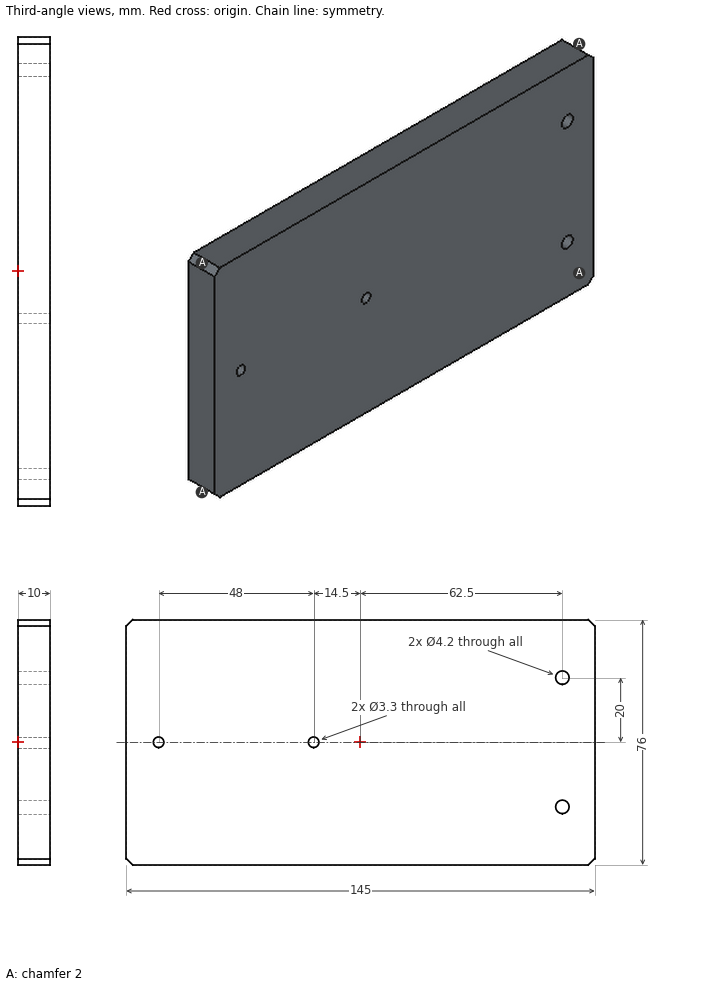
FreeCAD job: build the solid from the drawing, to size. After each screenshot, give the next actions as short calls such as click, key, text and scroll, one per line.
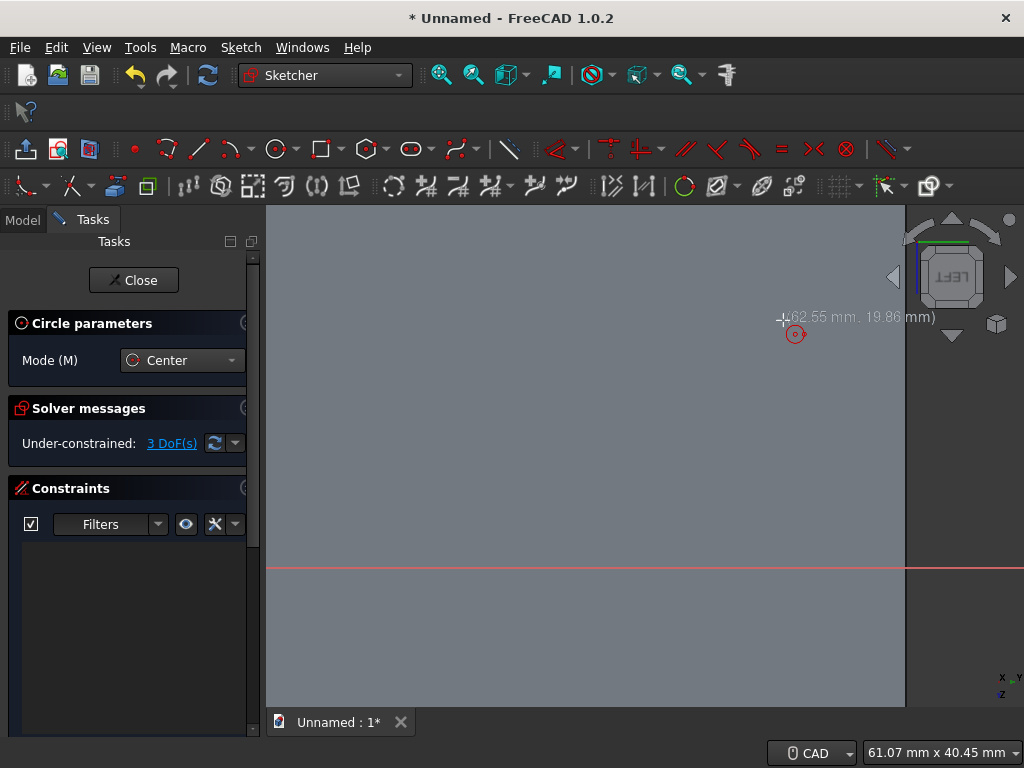
click(782, 320)
click(800, 301)
key(Escape)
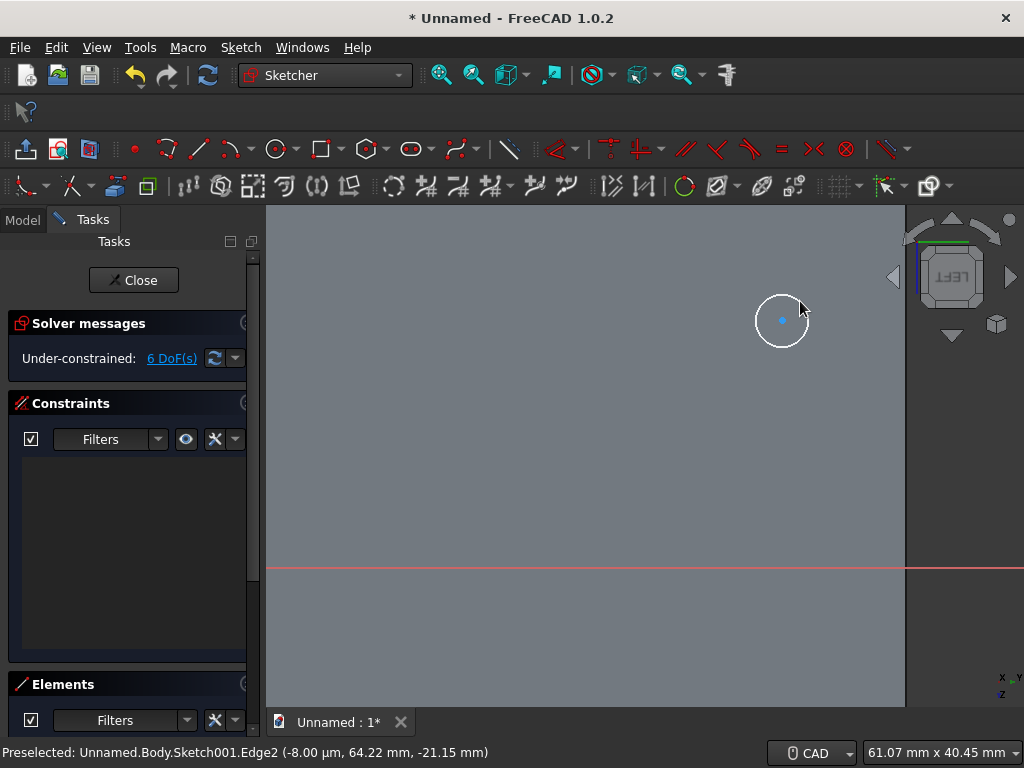
scroll(783, 320, down, 3)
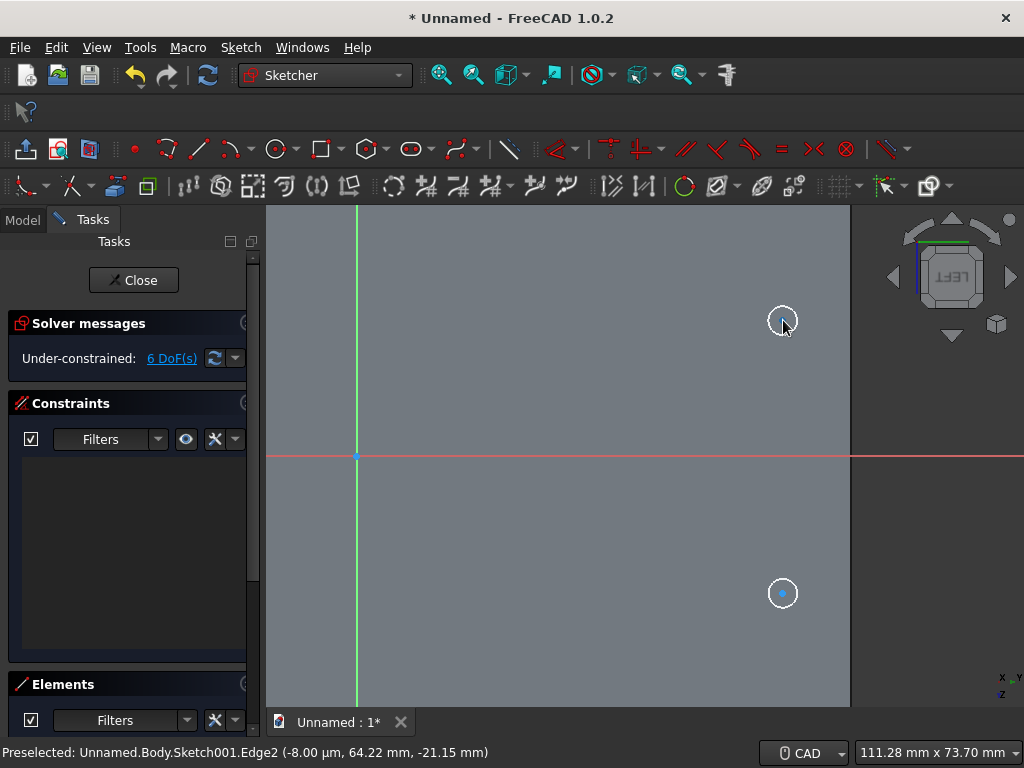
click(793, 583)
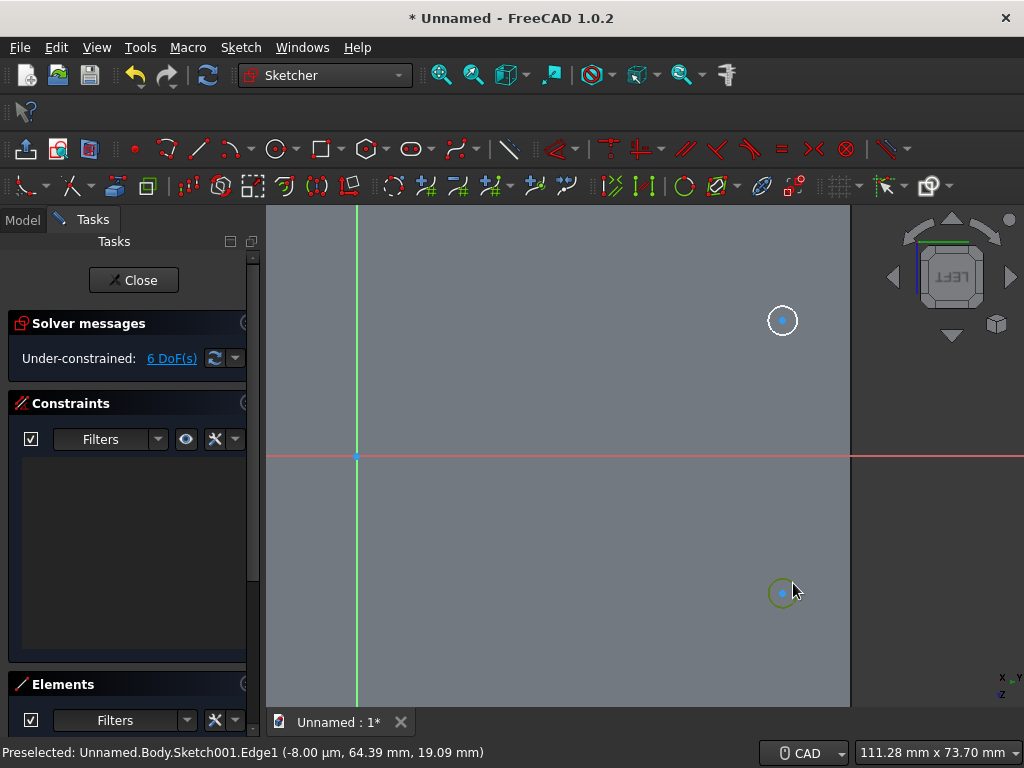
click(793, 310)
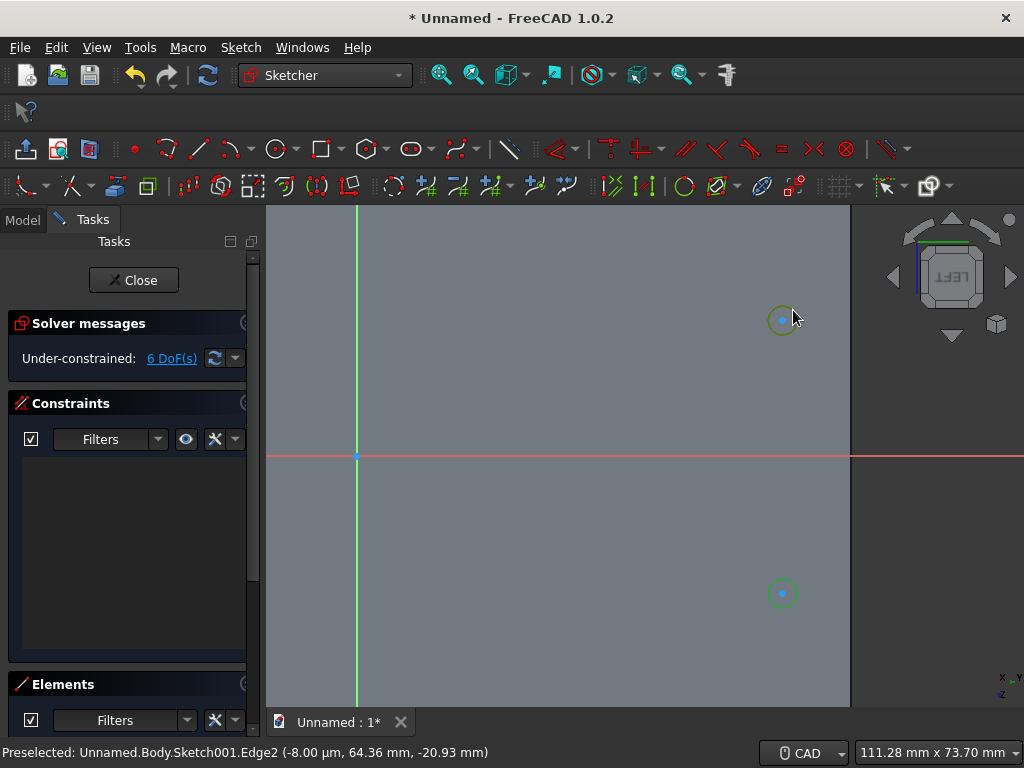
key(e)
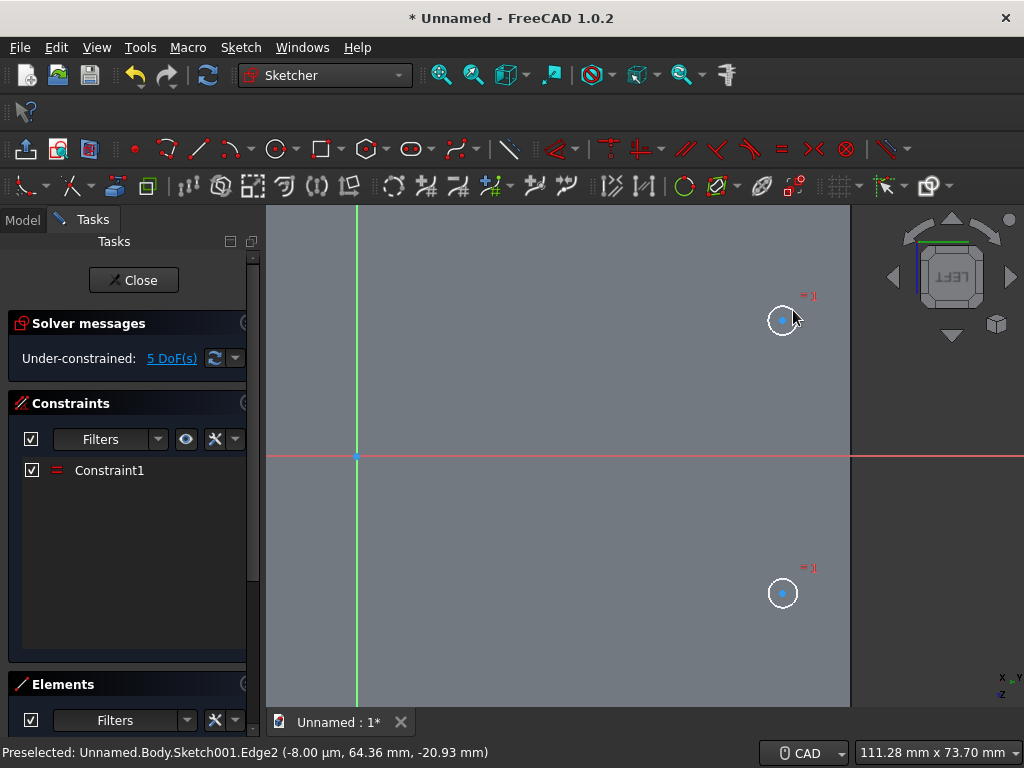
click(783, 593)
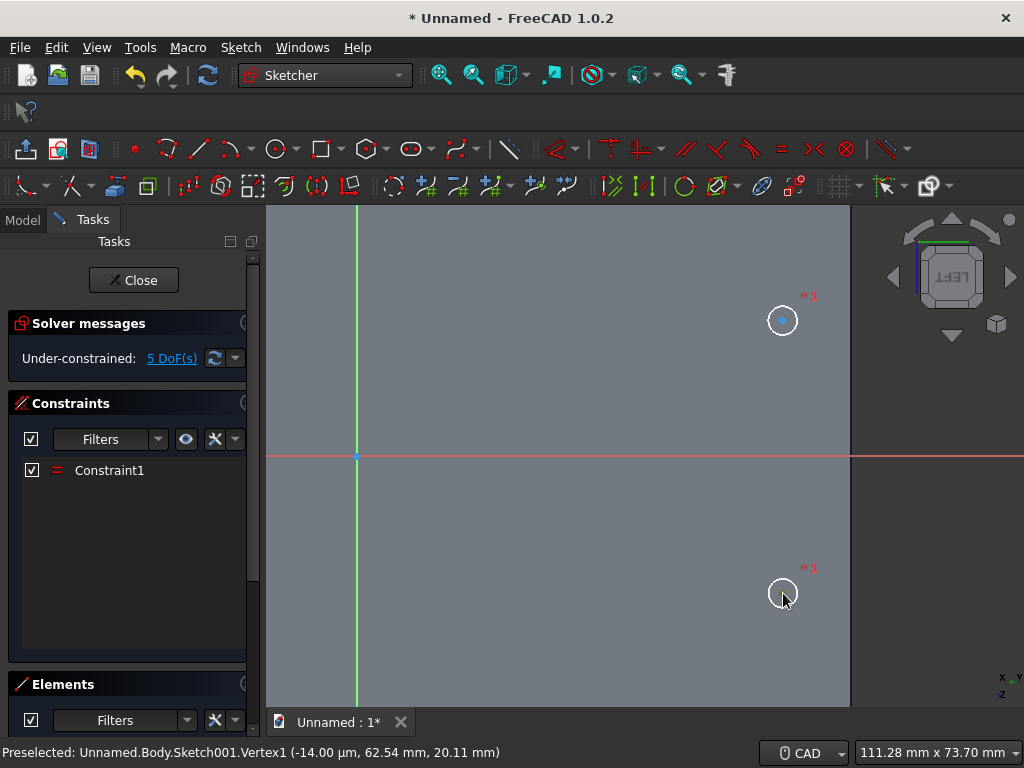
click(783, 321)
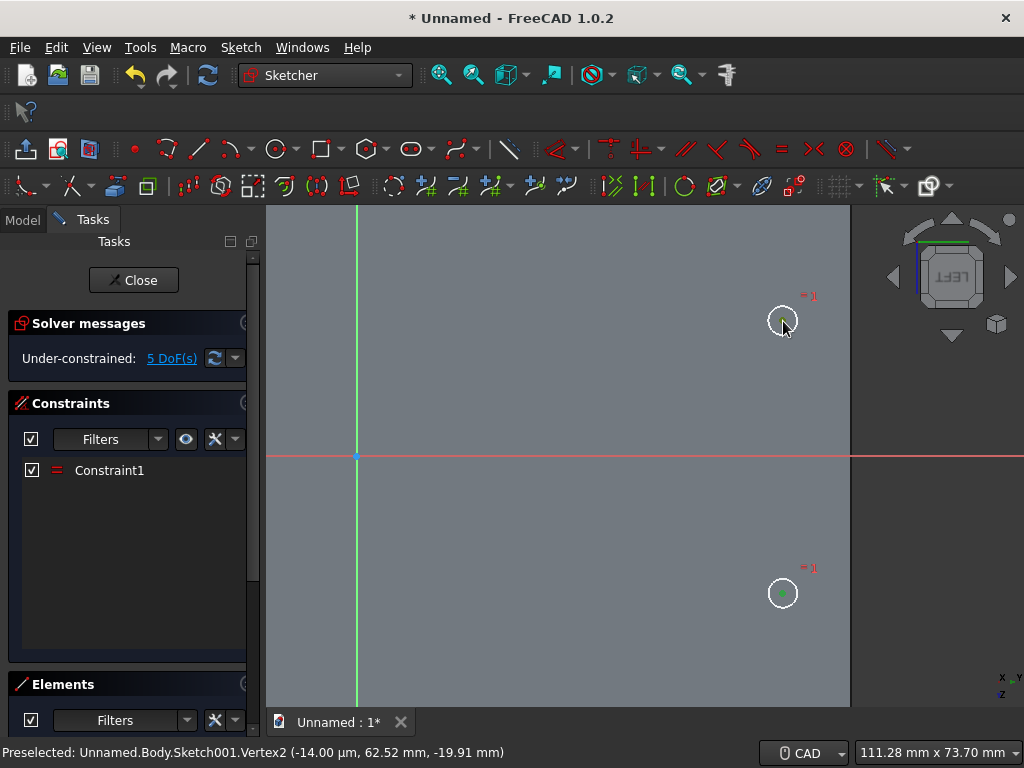
click(415, 456)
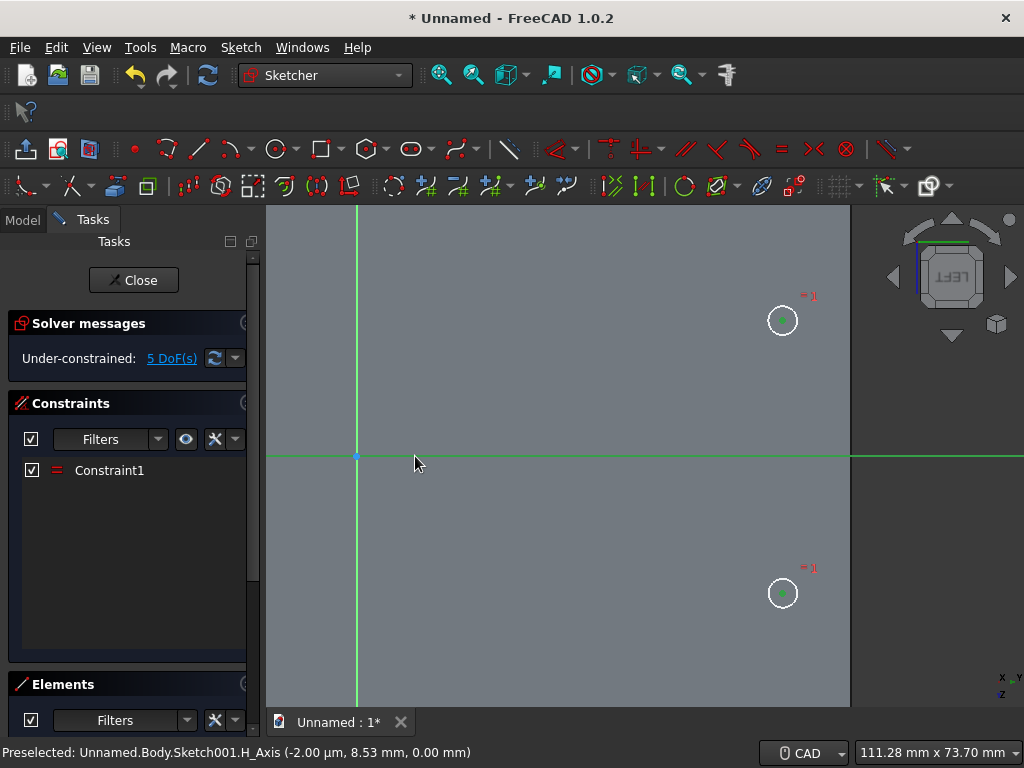
key(s)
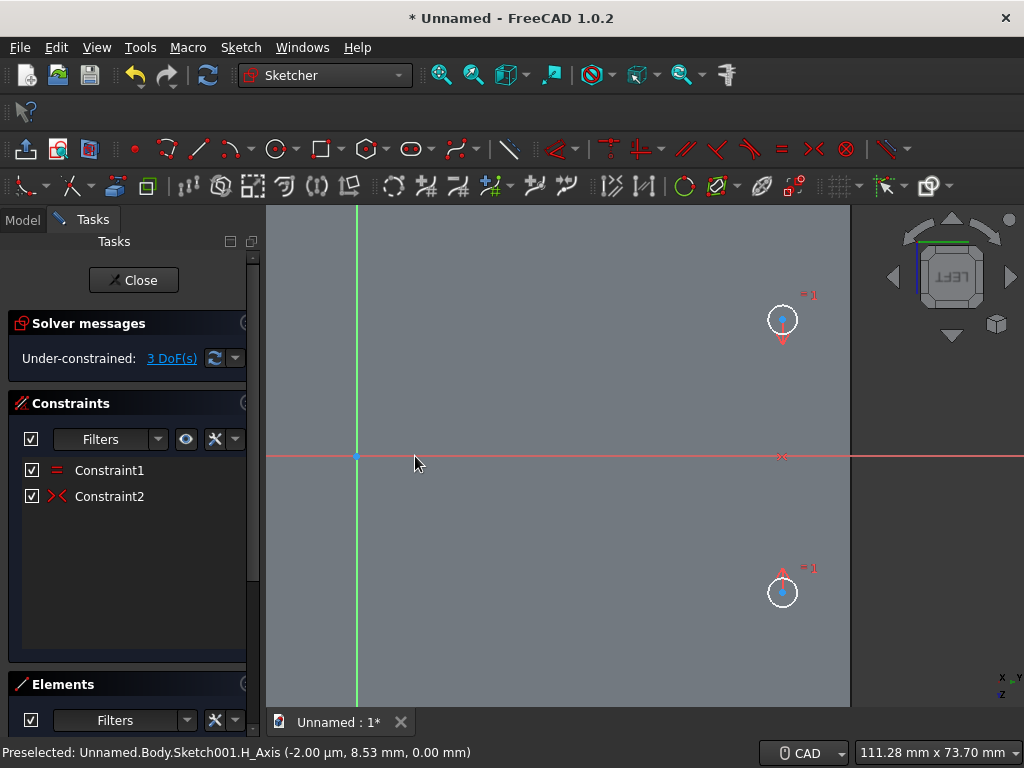
key(d)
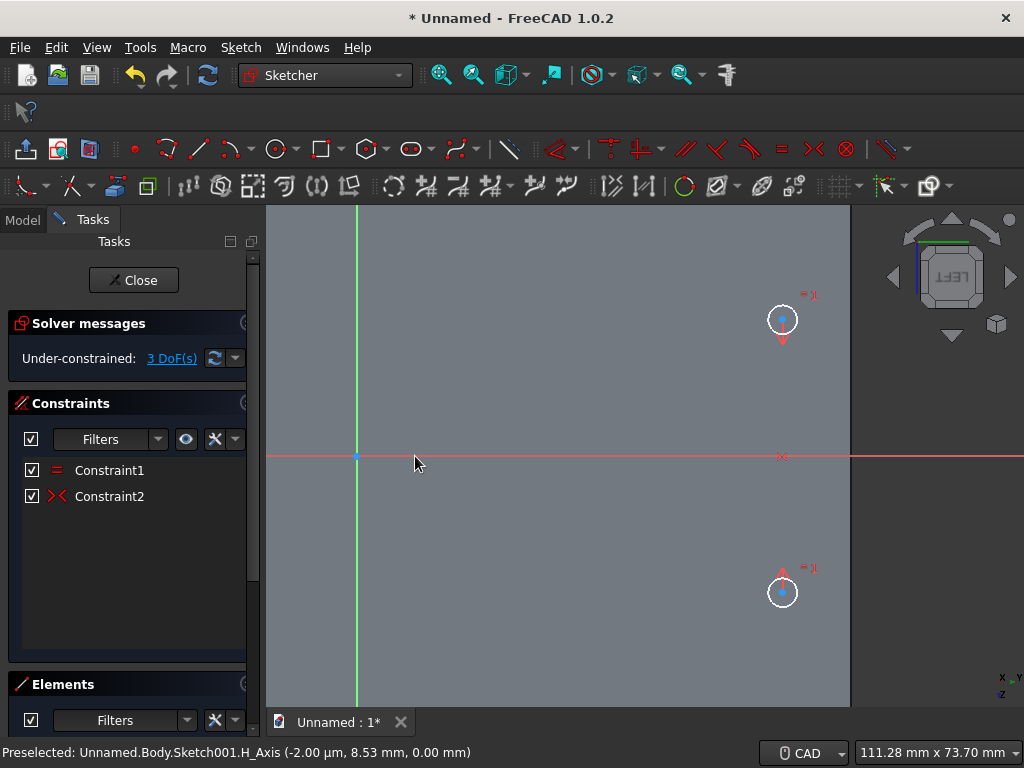
scroll(793, 583, up, 2)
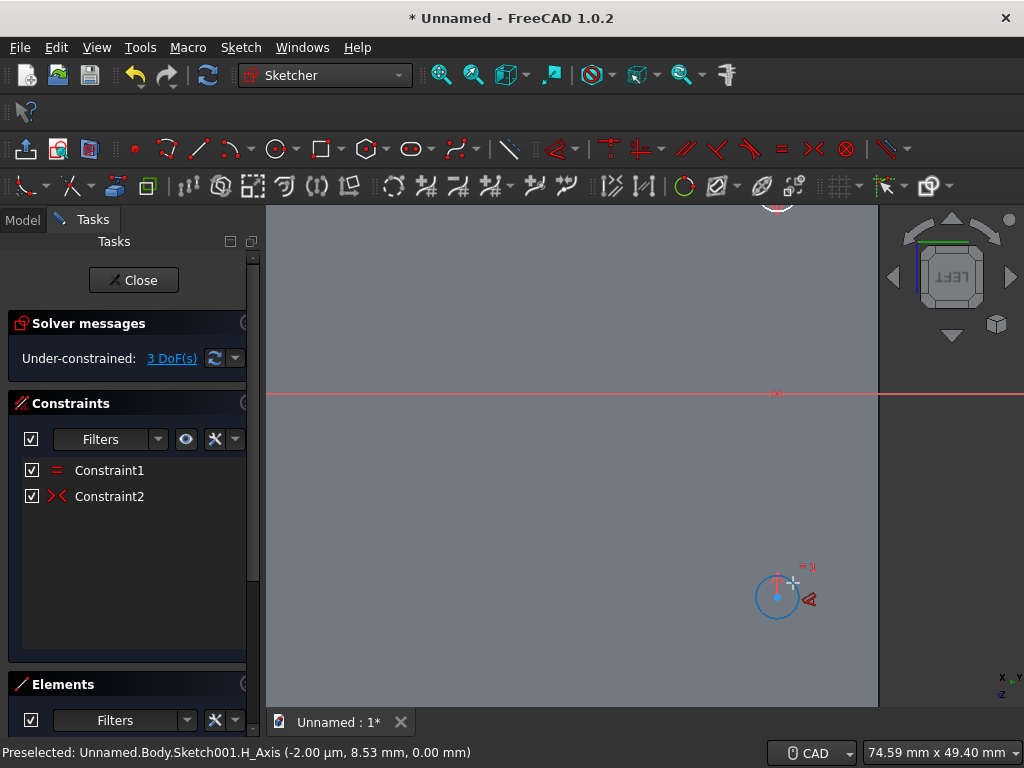
click(792, 582)
click(814, 559)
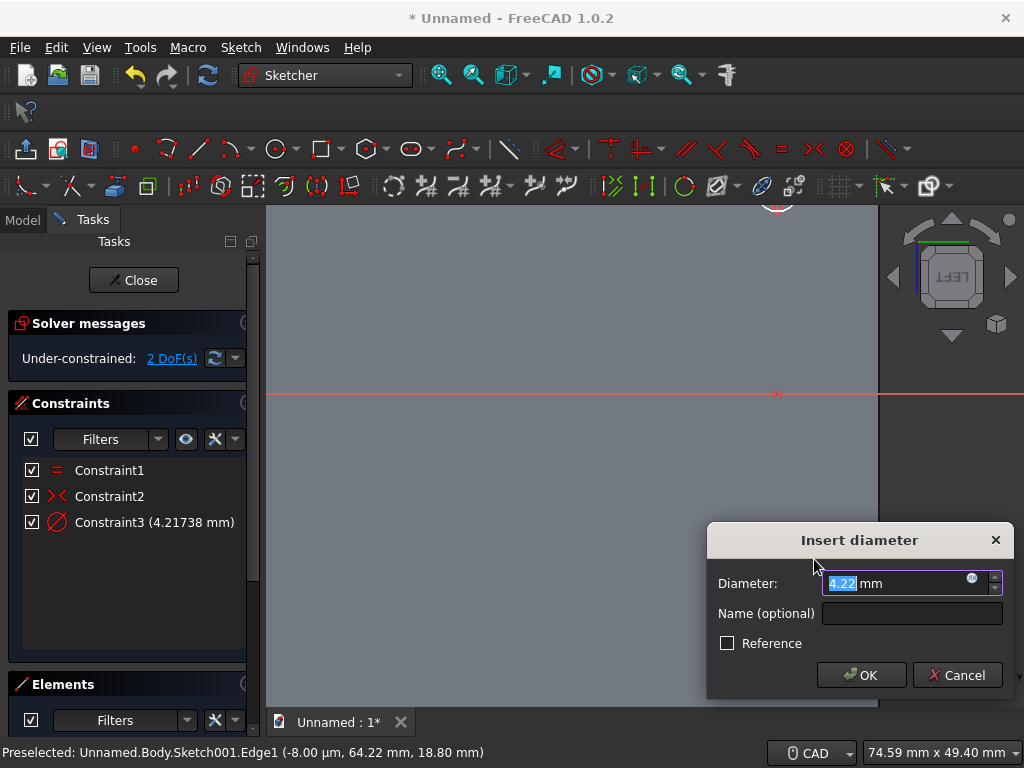
text(4.2)
key(Return)